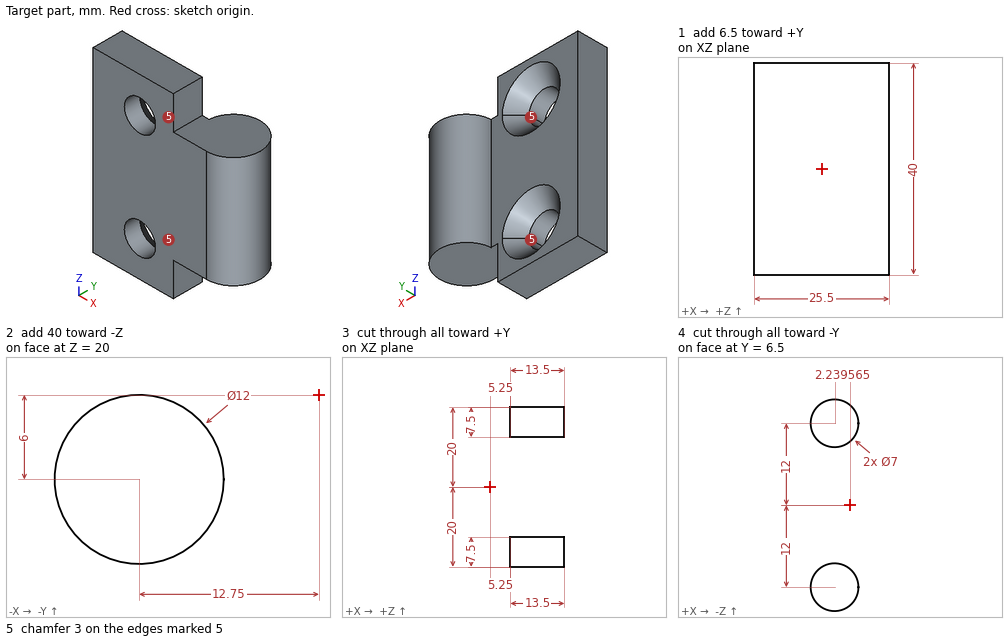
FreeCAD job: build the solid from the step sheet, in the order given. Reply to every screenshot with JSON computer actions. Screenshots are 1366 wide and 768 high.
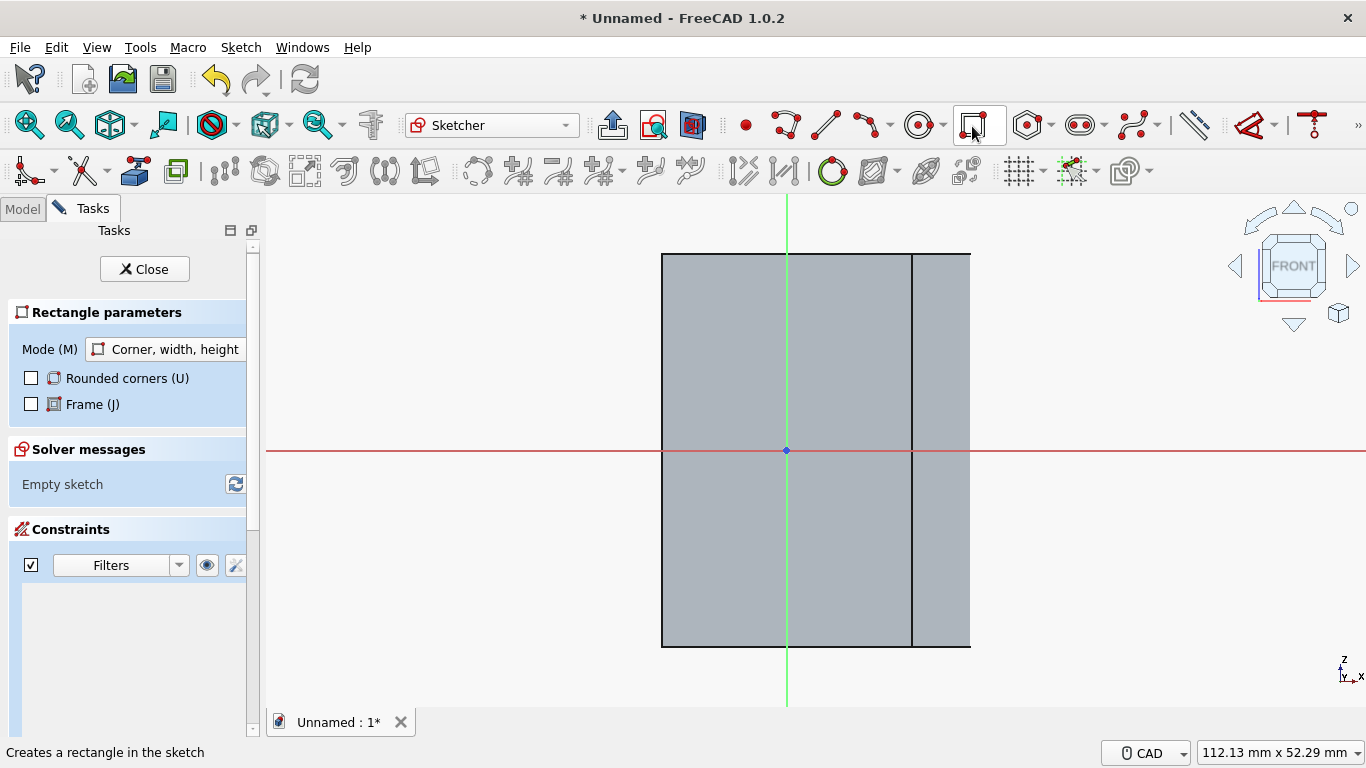
{"action": "left_click", "coordinate": [838, 254]}
{"action": "left_click", "coordinate": [971, 328]}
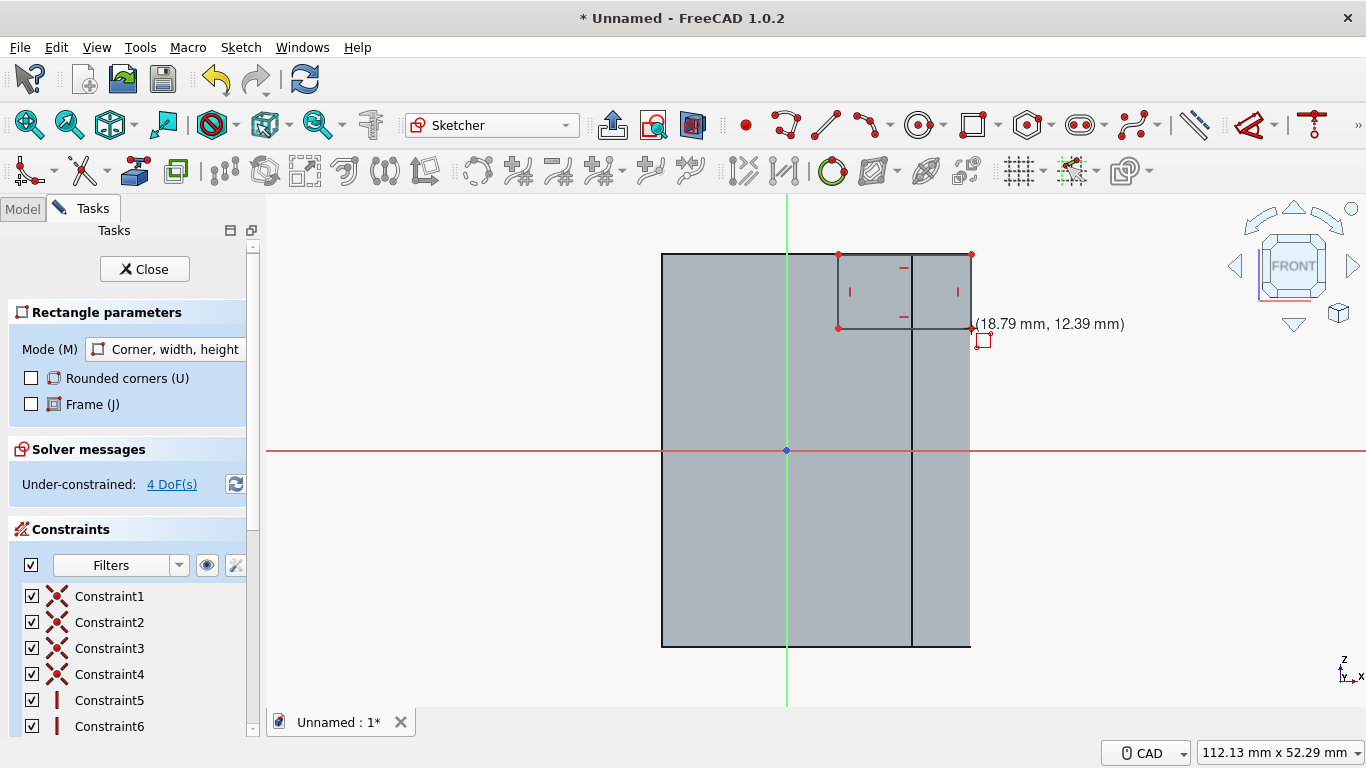
{"action": "left_click", "coordinate": [838, 573]}
{"action": "left_click", "coordinate": [971, 647]}
{"action": "key", "text": "Escape"}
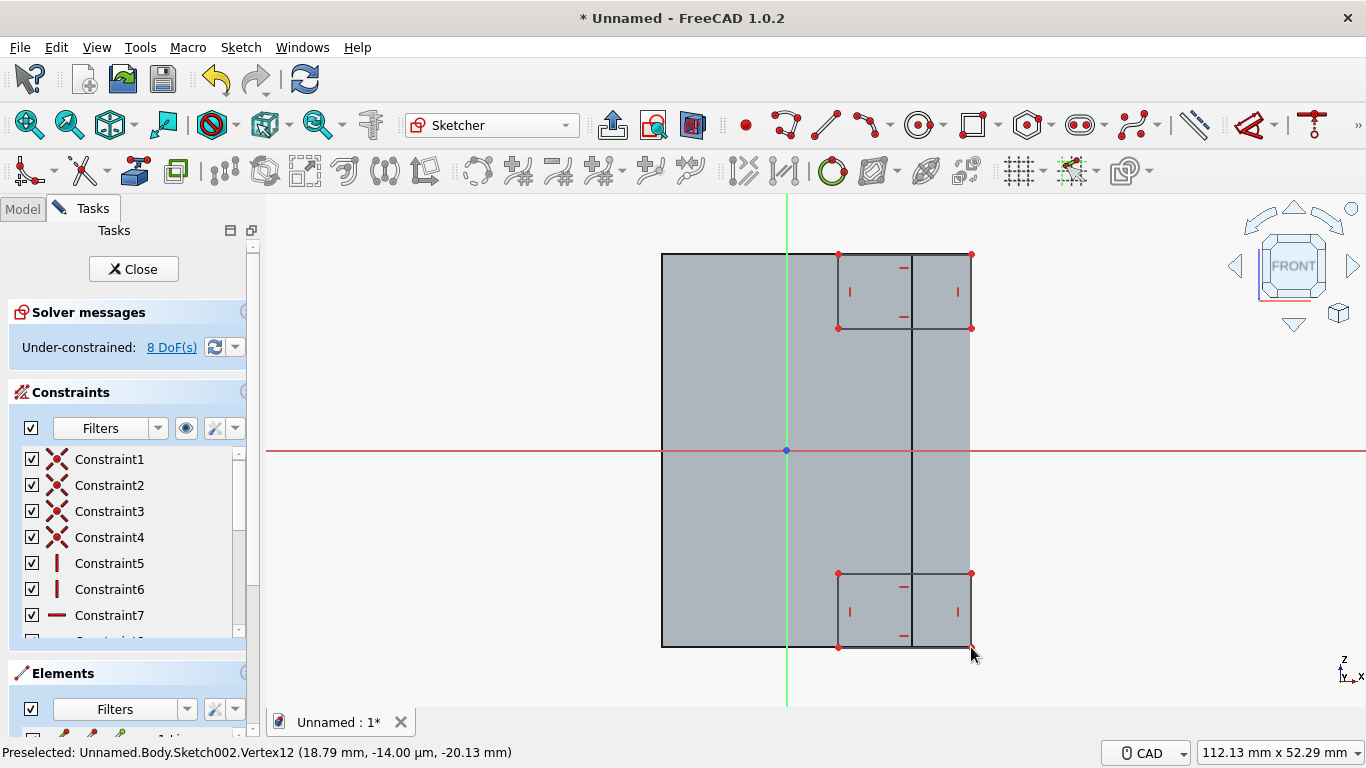
{"action": "left_click", "coordinate": [1250, 126]}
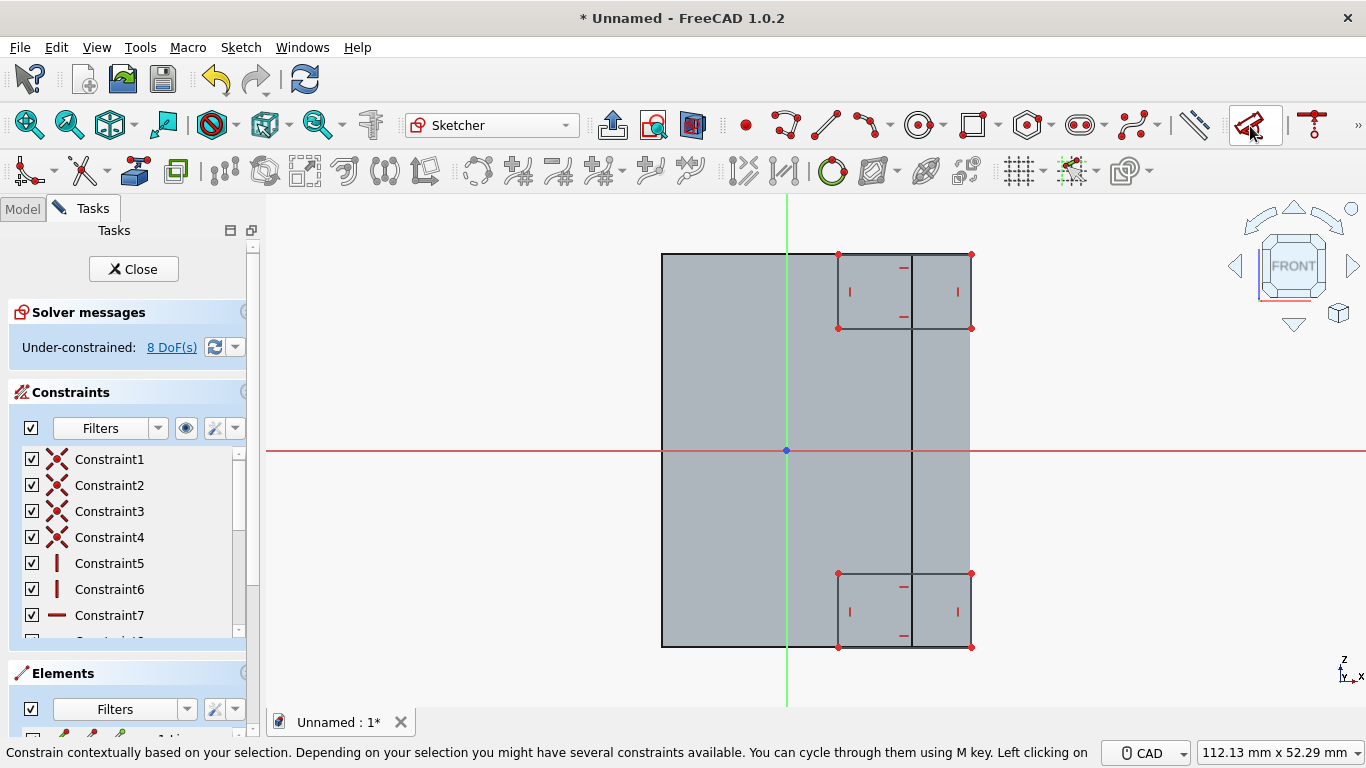
{"action": "left_click", "coordinate": [838, 277]}
{"action": "left_click", "coordinate": [804, 292]}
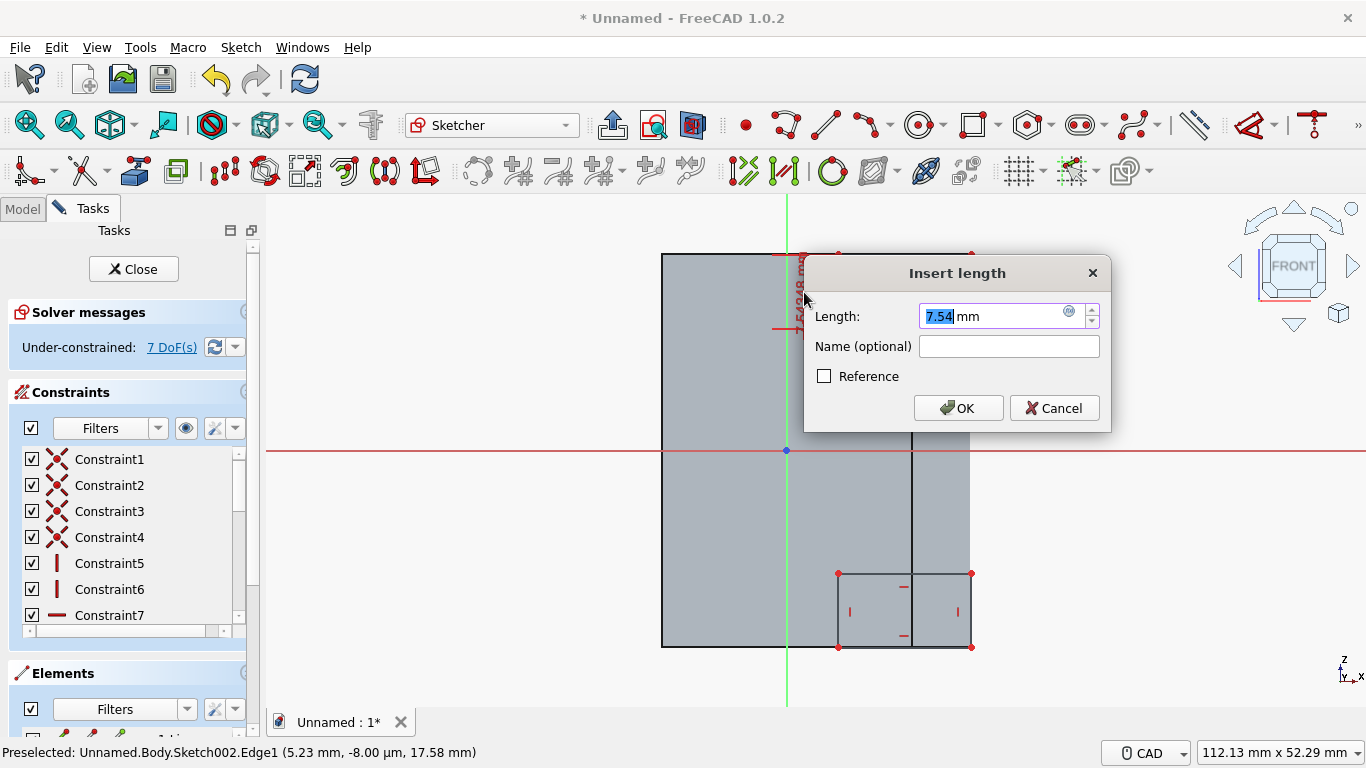
{"action": "type", "text": "7.5"}
{"action": "key", "text": "Return"}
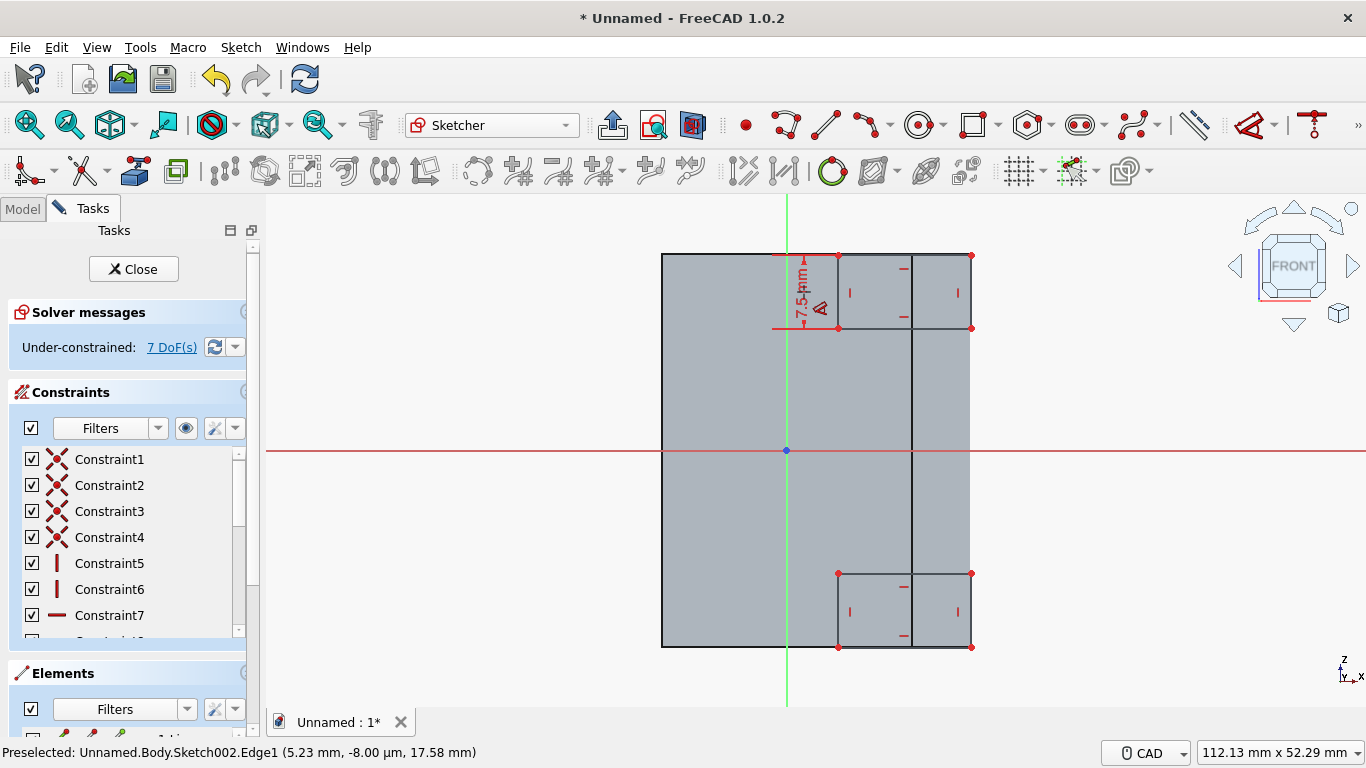
{"action": "left_click", "coordinate": [838, 596]}
{"action": "left_click", "coordinate": [804, 611]}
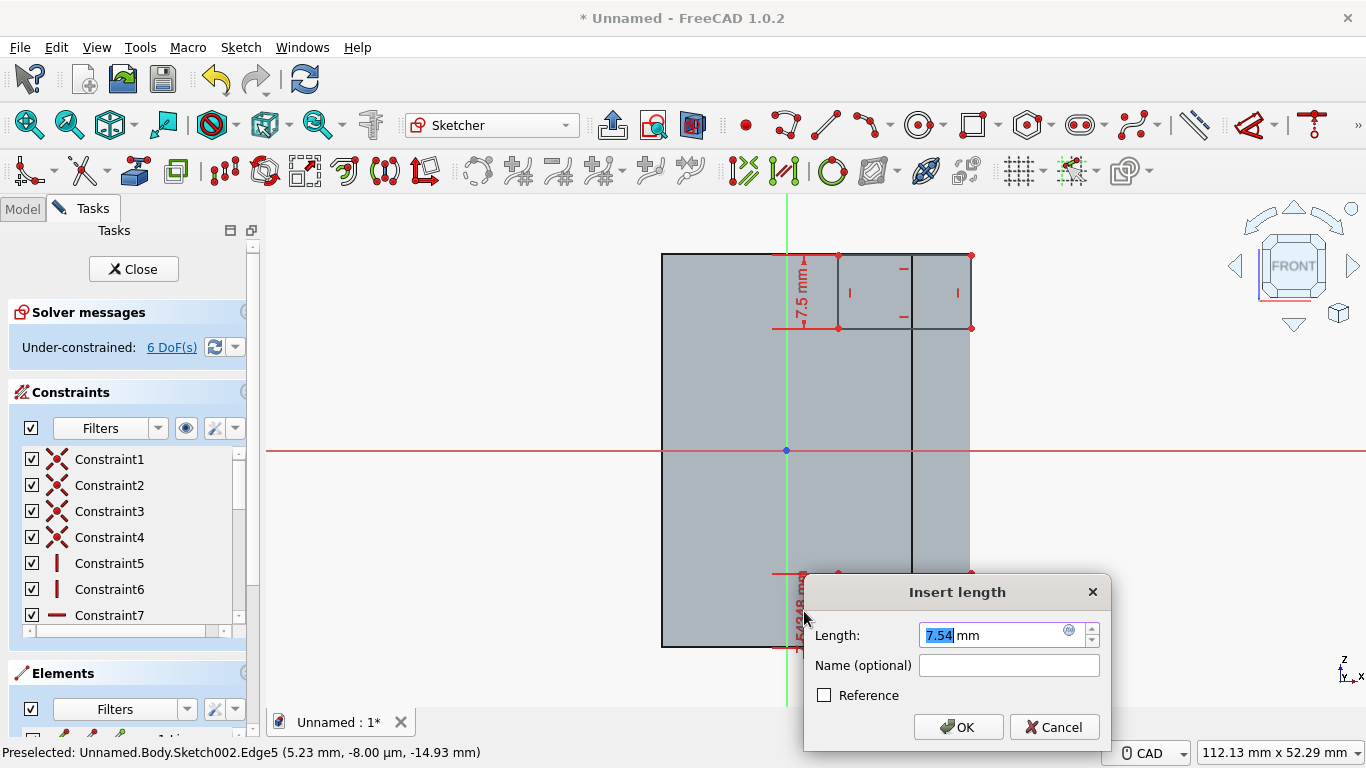
{"action": "type", "text": "7.5"}
{"action": "key", "text": "Return"}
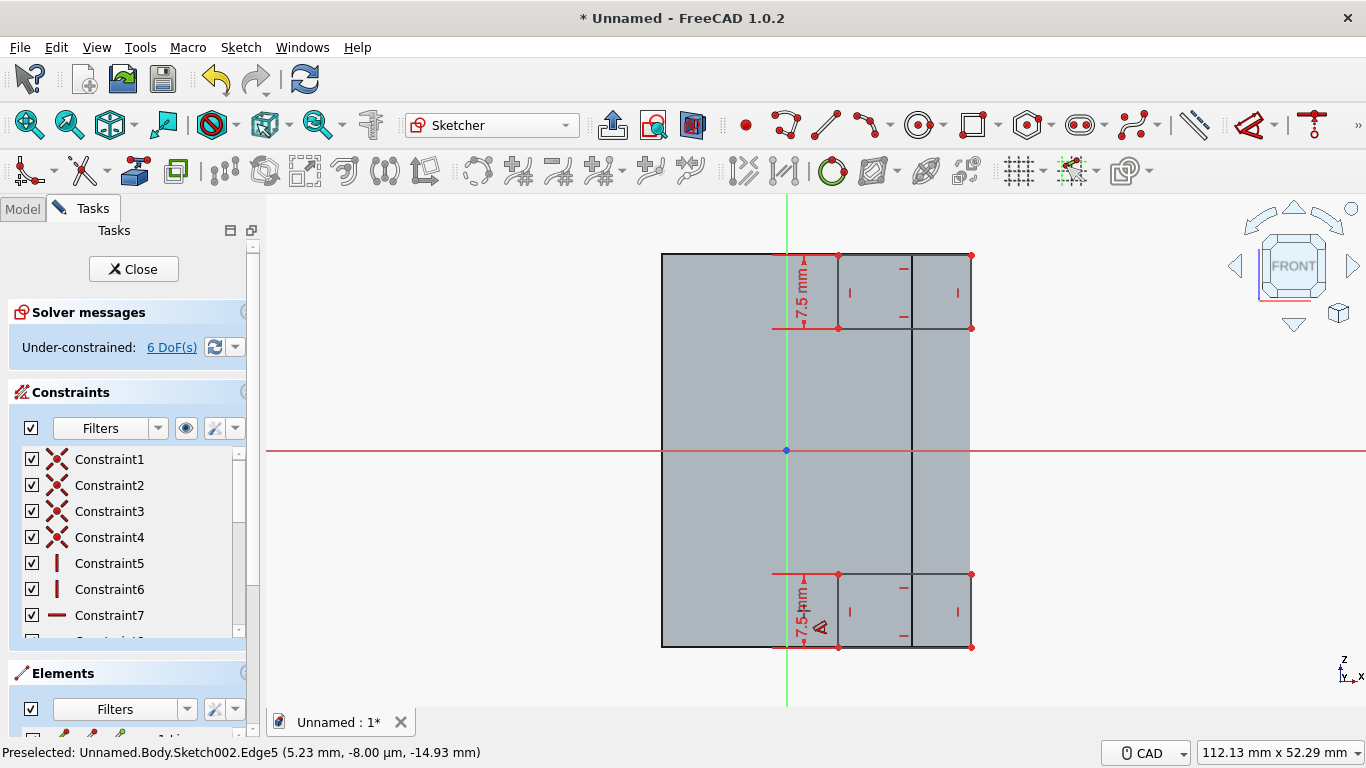
{"action": "left_click", "coordinate": [838, 255]}
{"action": "left_click", "coordinate": [753, 353]}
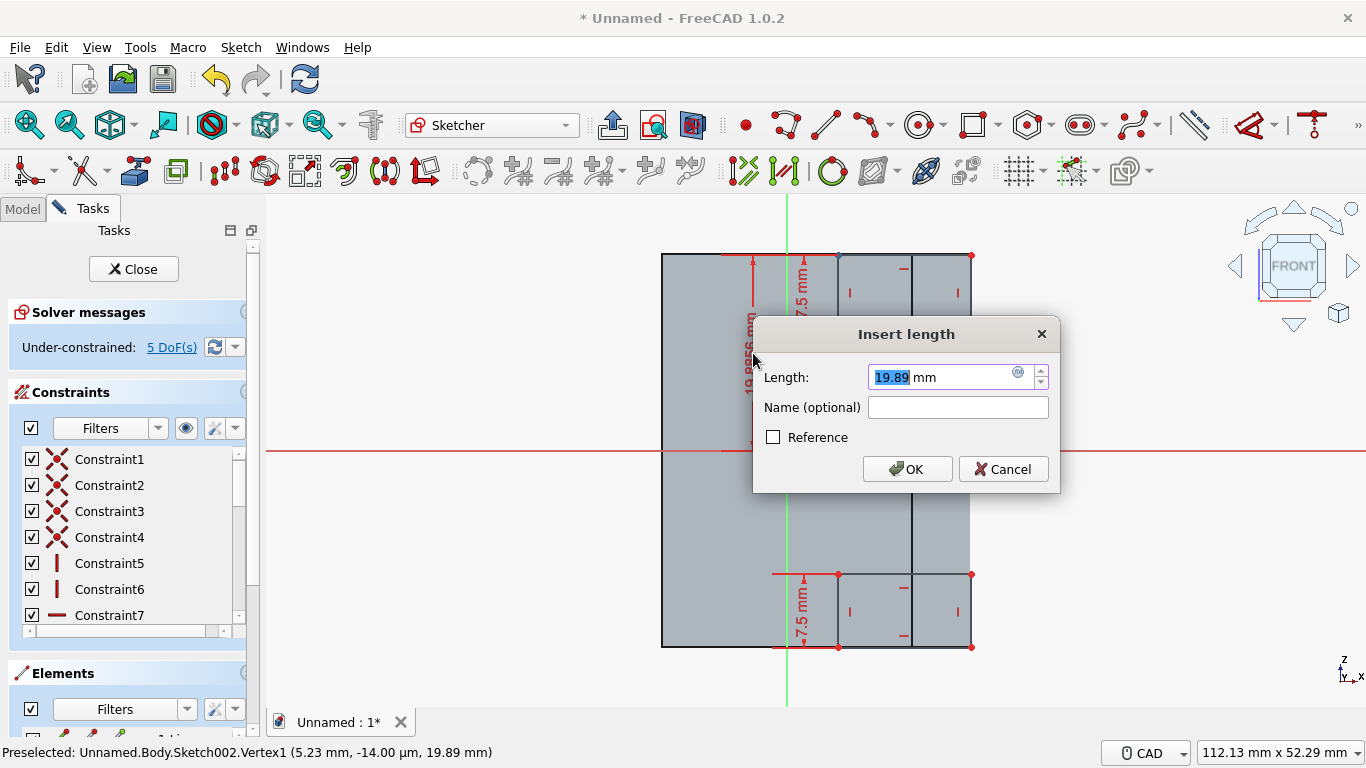
{"action": "type", "text": "20"}
{"action": "key", "text": "Return"}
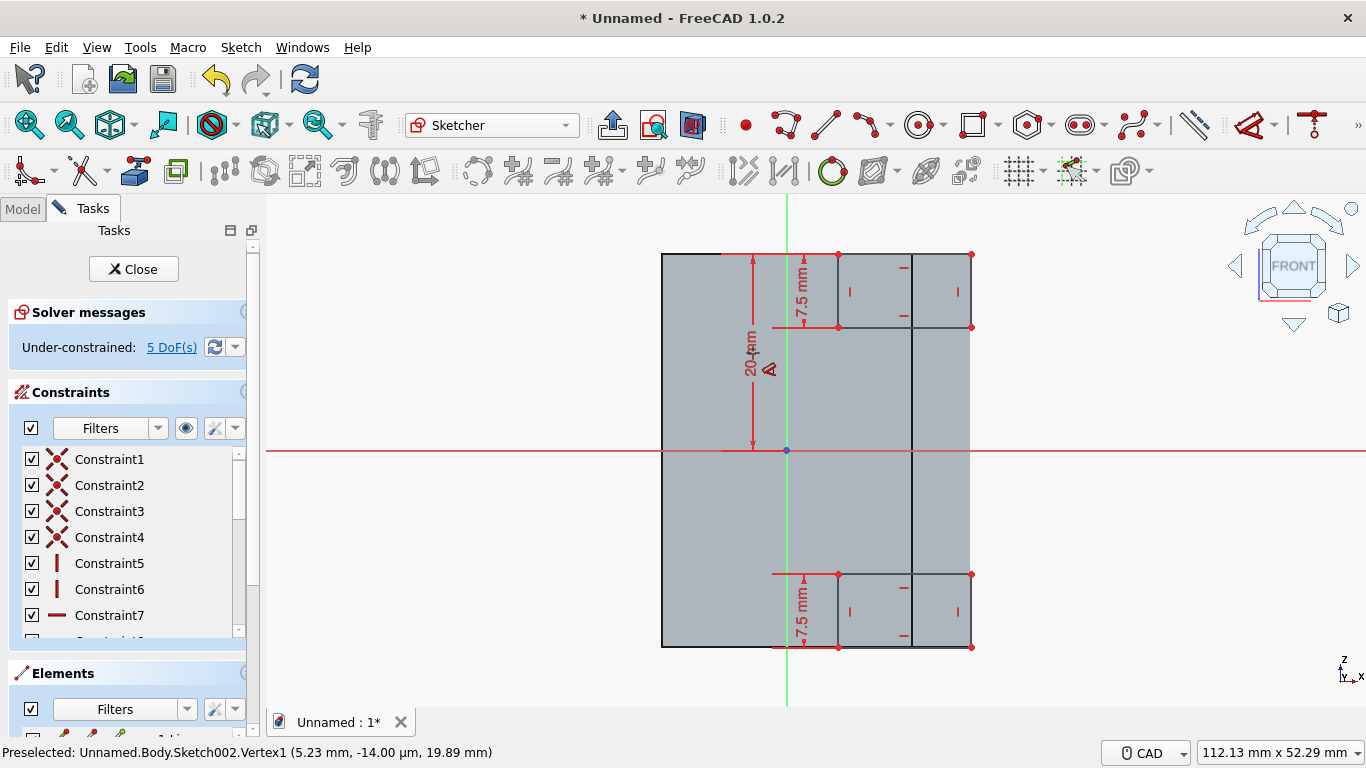
{"action": "left_click", "coordinate": [838, 648]}
{"action": "left_click", "coordinate": [753, 549]}